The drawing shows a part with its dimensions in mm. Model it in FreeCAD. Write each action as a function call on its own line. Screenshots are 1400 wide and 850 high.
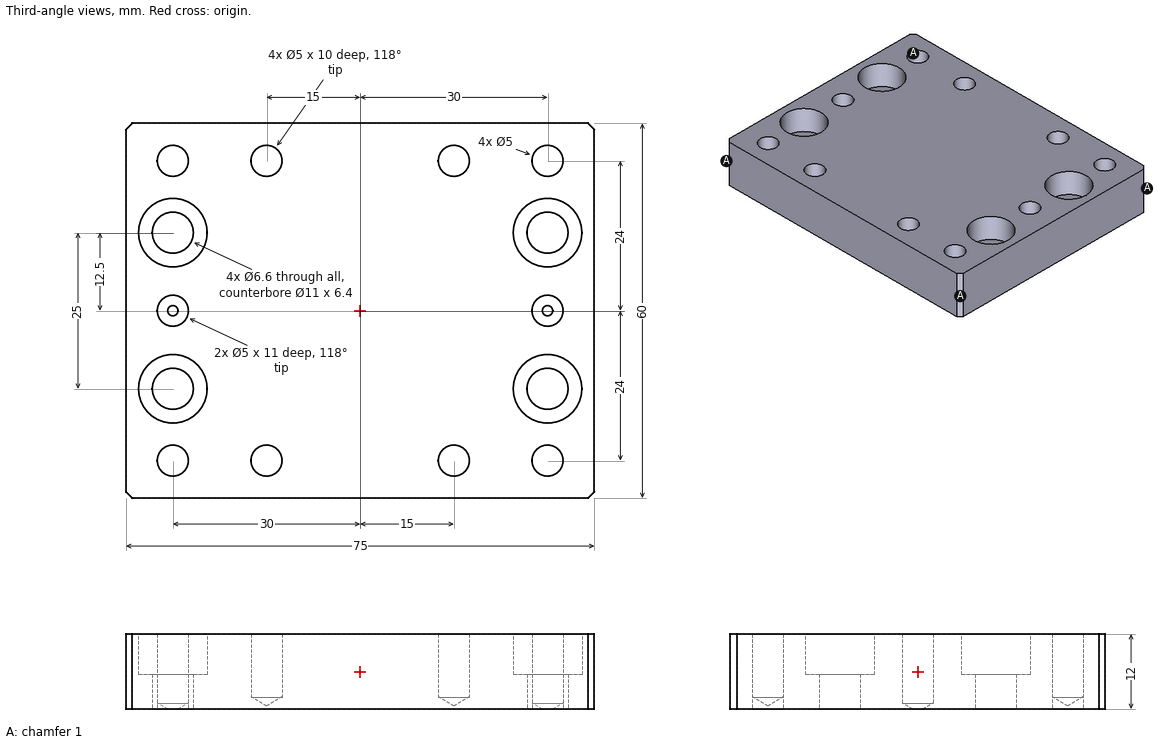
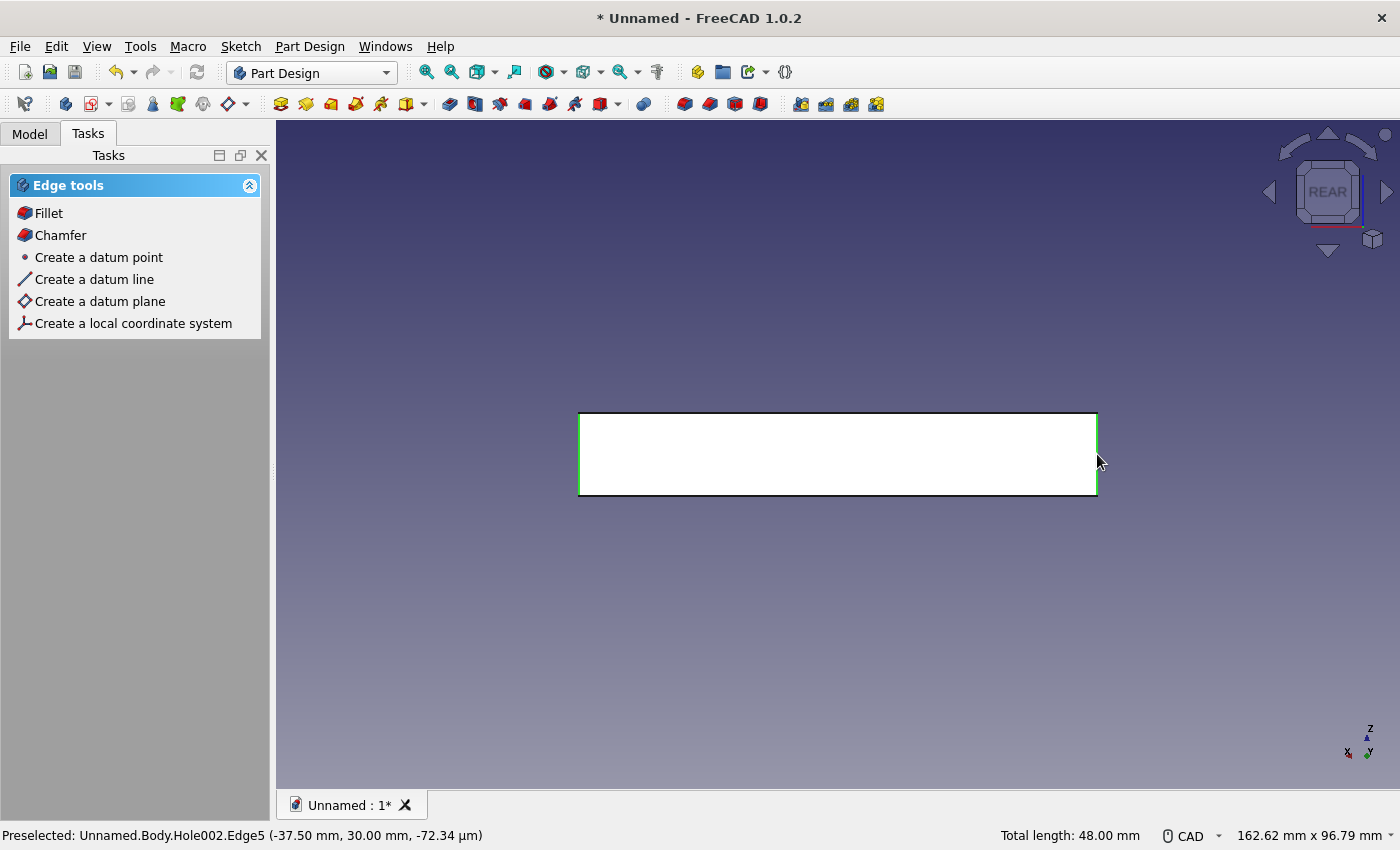
click(710, 104)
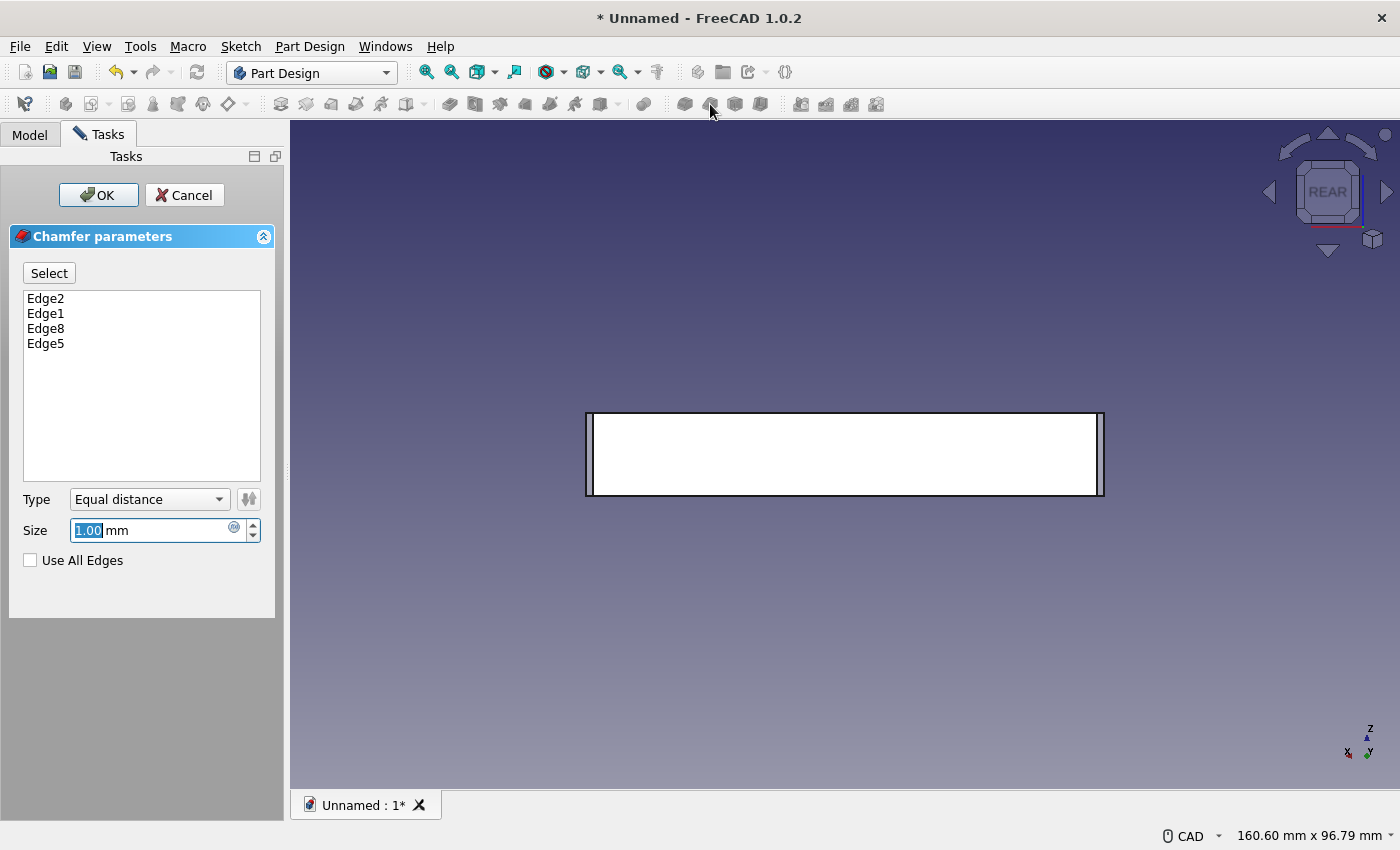
text(1)
key(Tab)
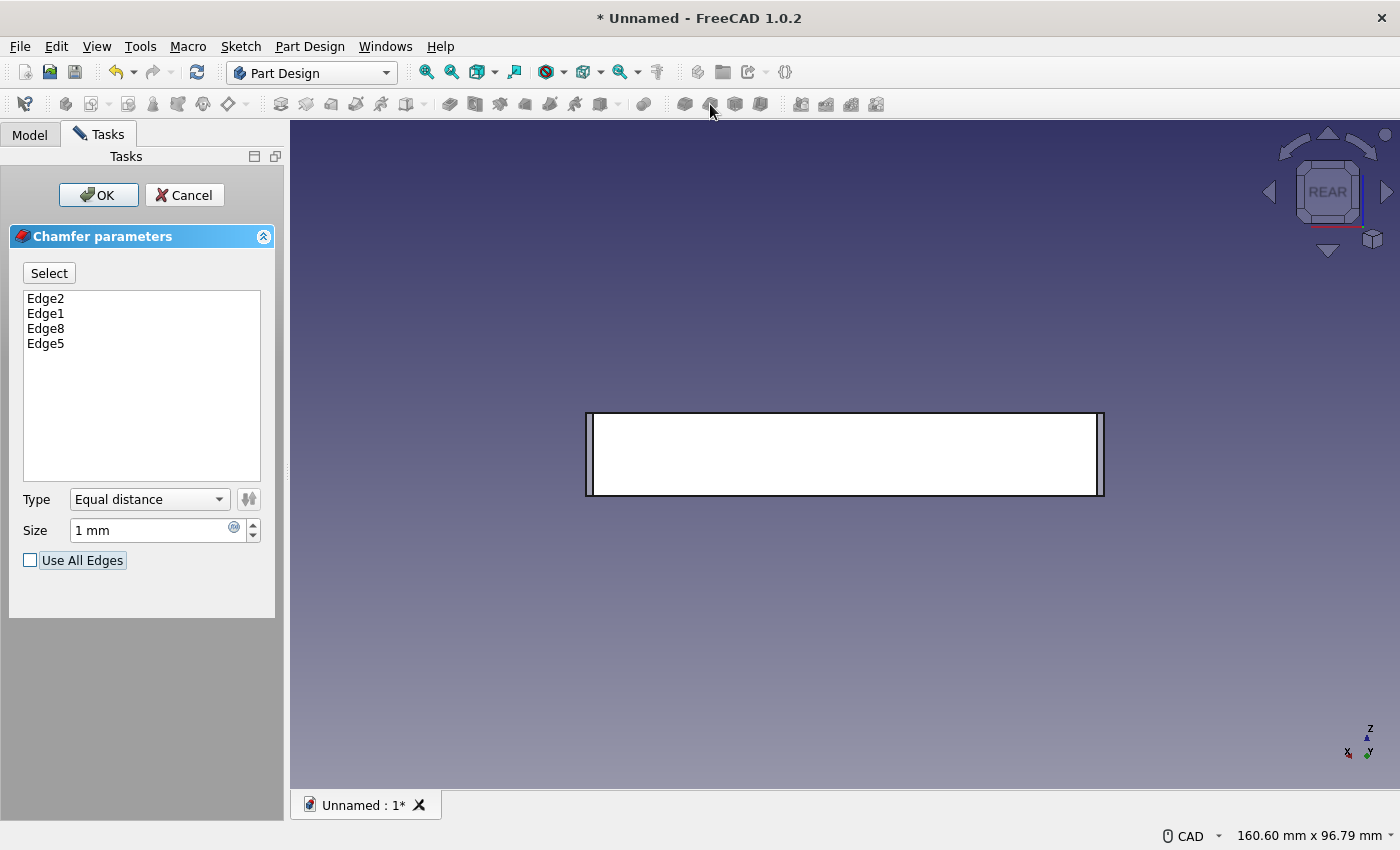
click(99, 195)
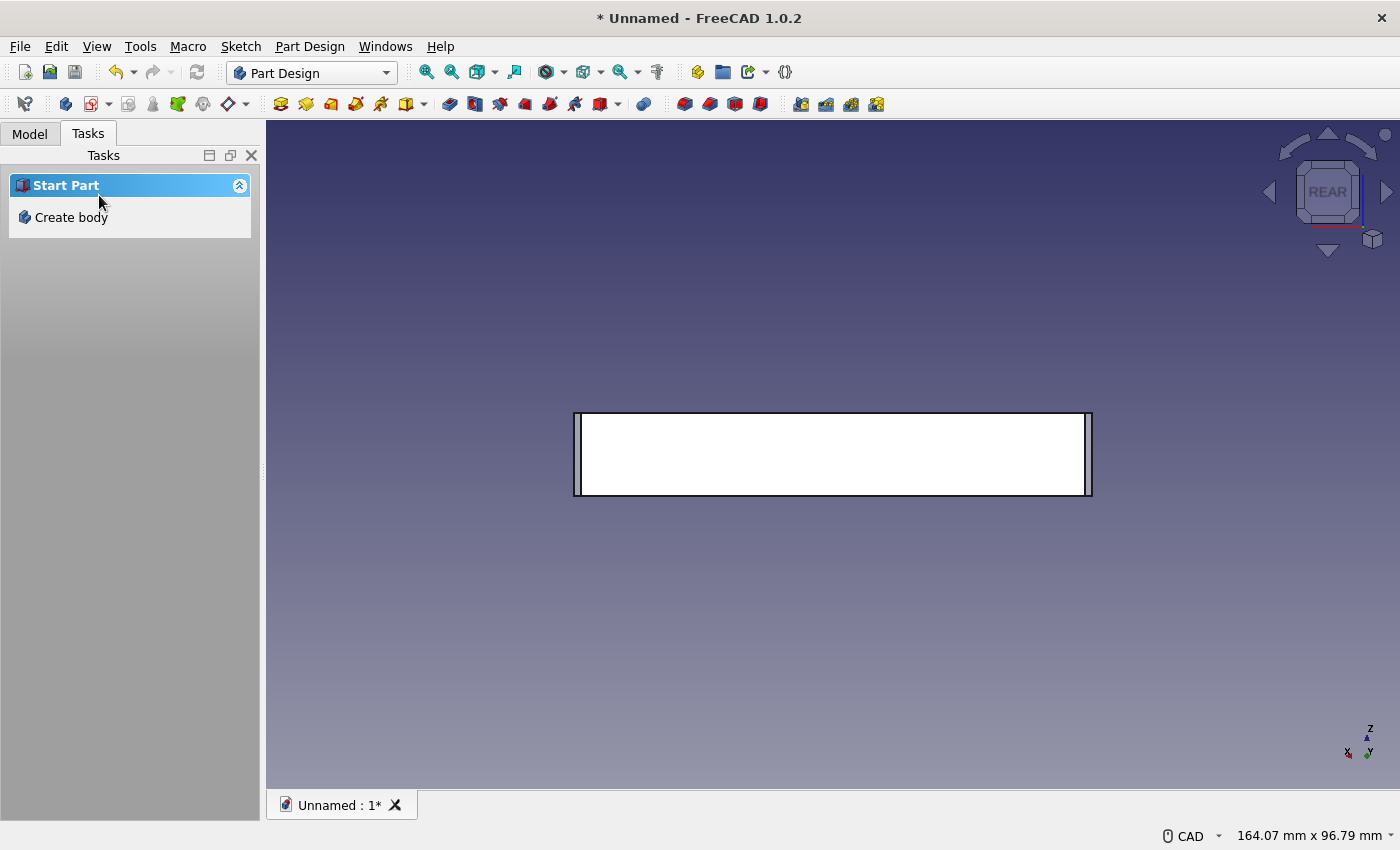
key(0)